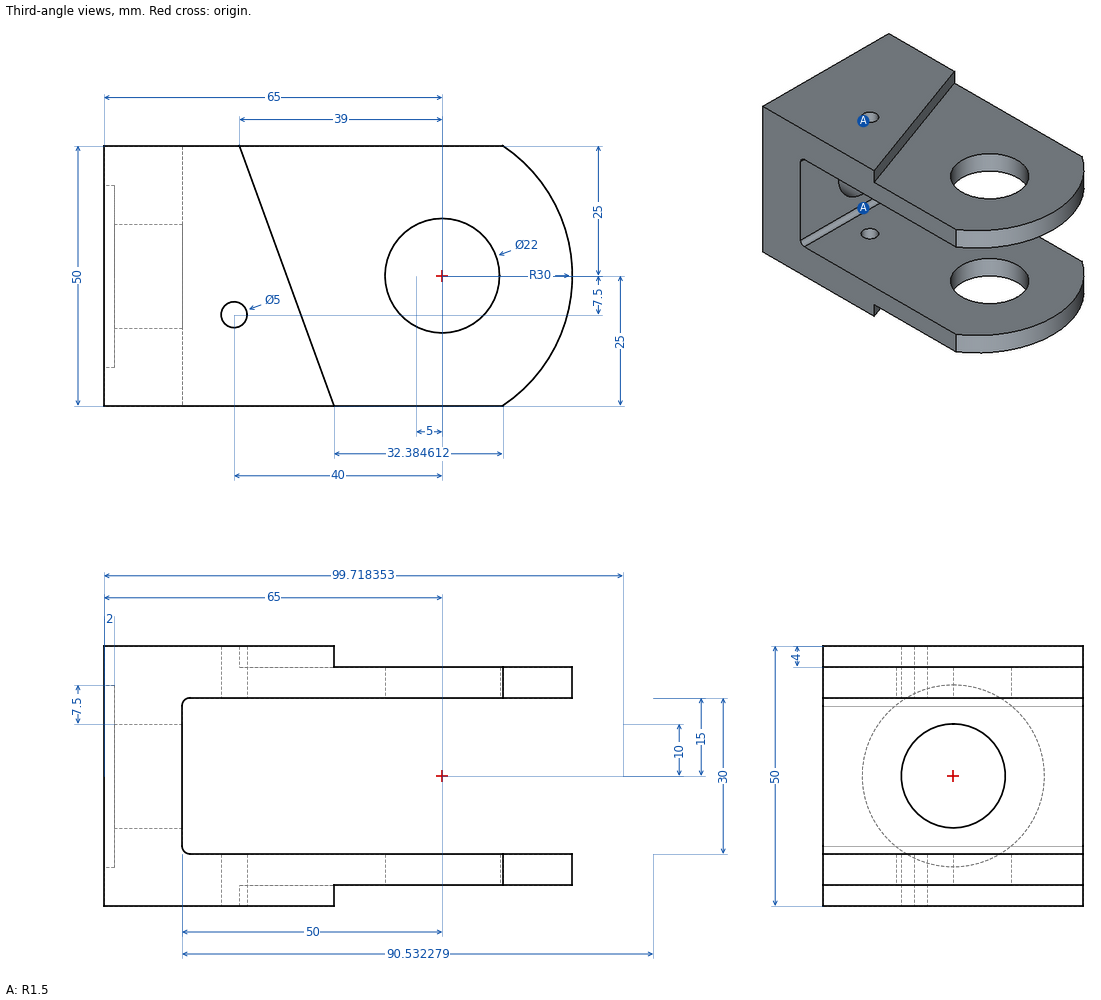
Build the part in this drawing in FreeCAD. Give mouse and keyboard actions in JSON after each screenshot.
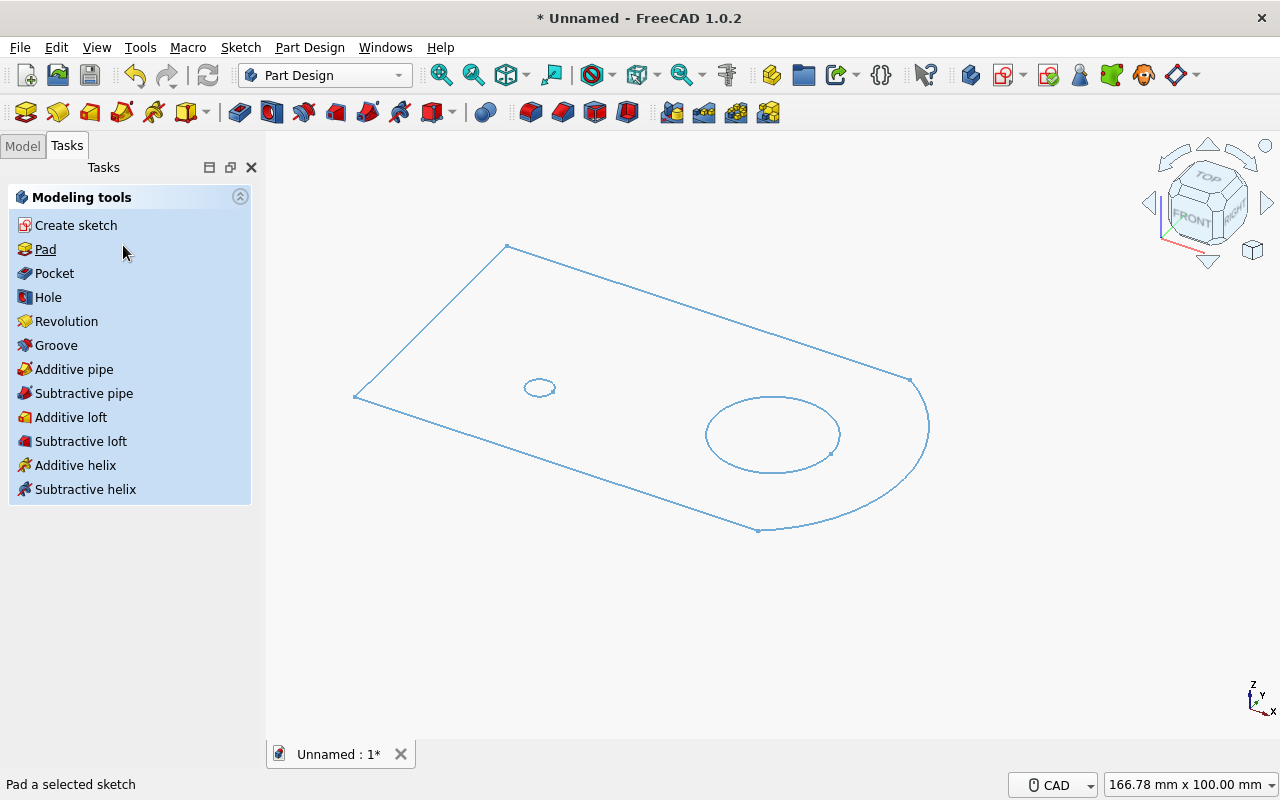
{"action": "left_click", "coordinate": [26, 112]}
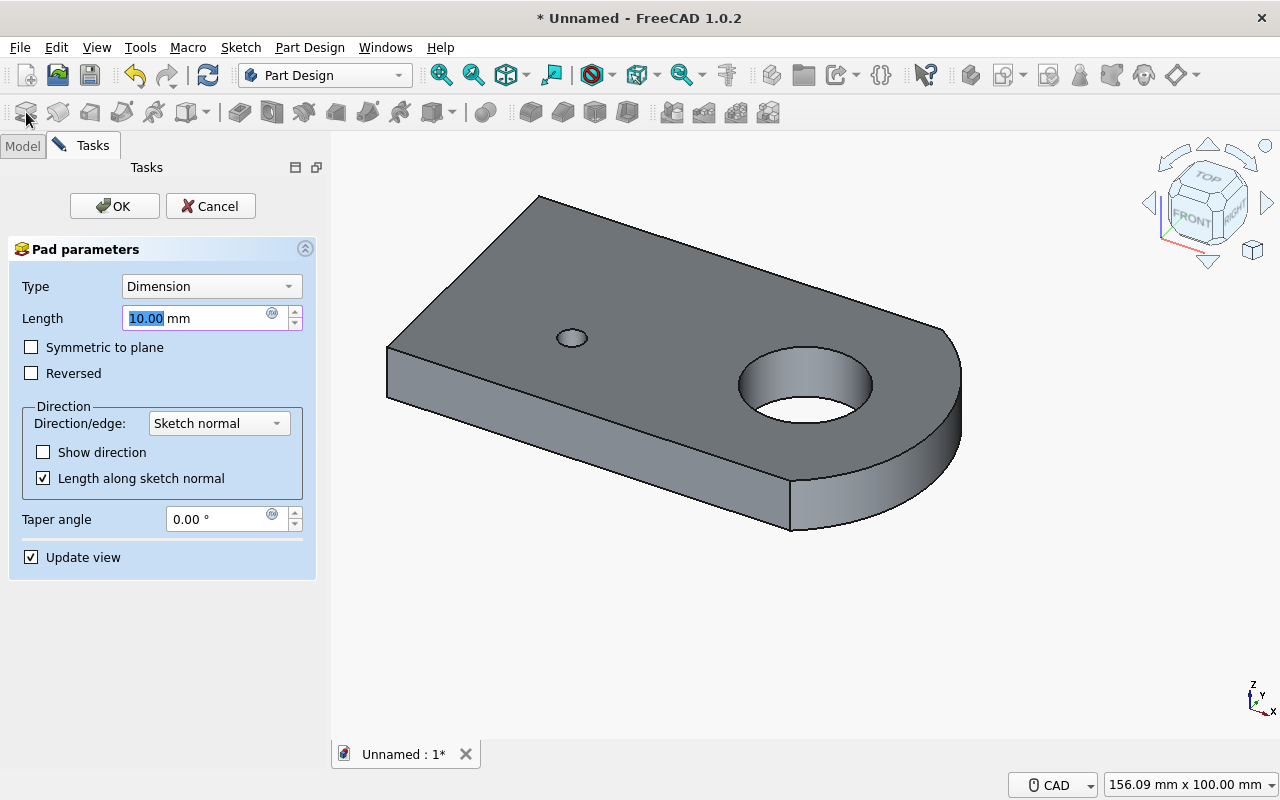
{"action": "type", "text": "50"}
{"action": "key", "text": "Tab"}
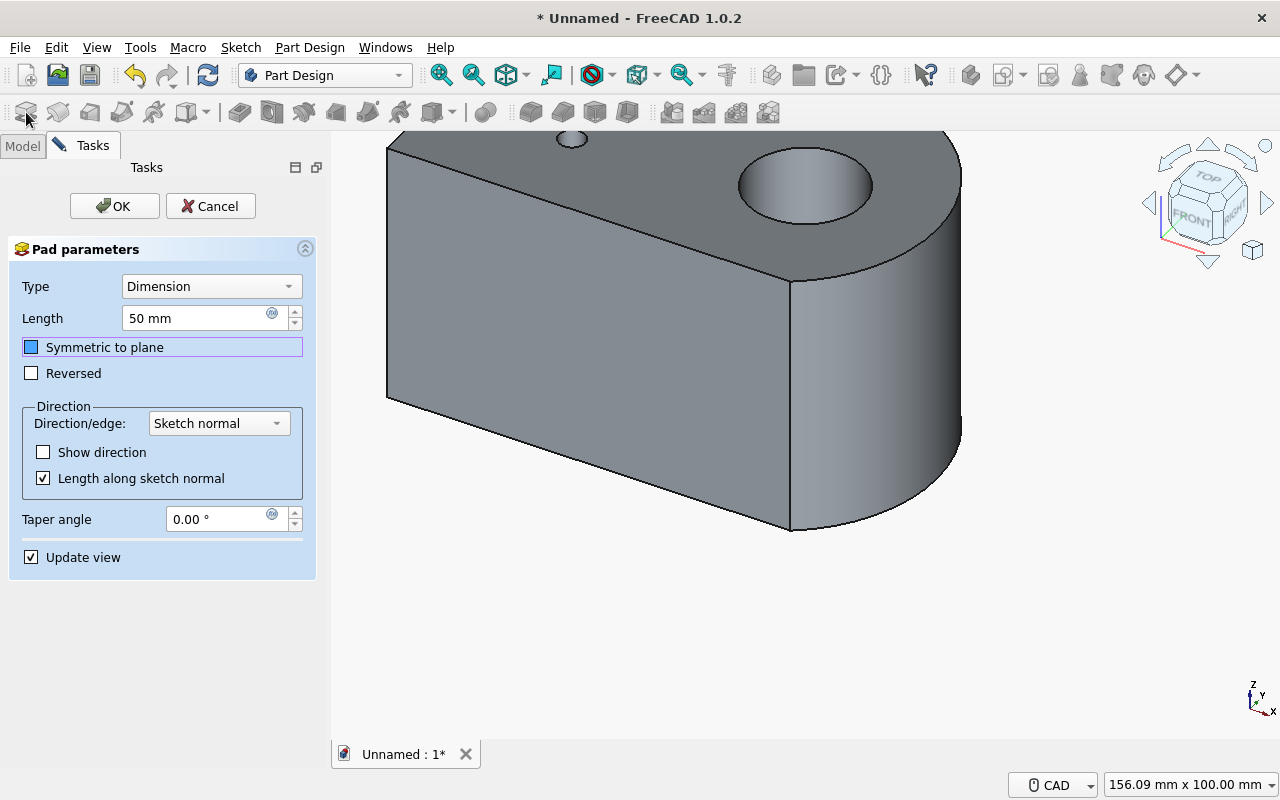
{"action": "left_click", "coordinate": [30, 347]}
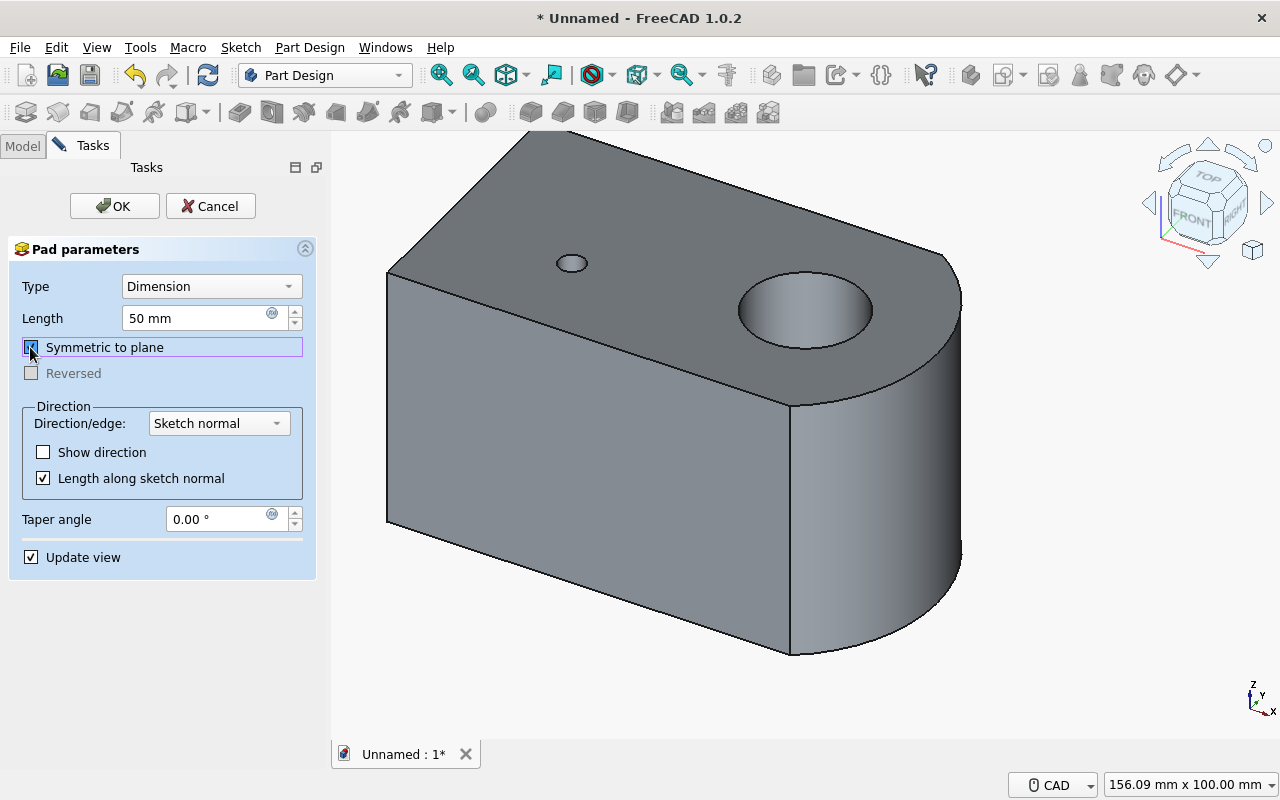
{"action": "left_click", "coordinate": [115, 206]}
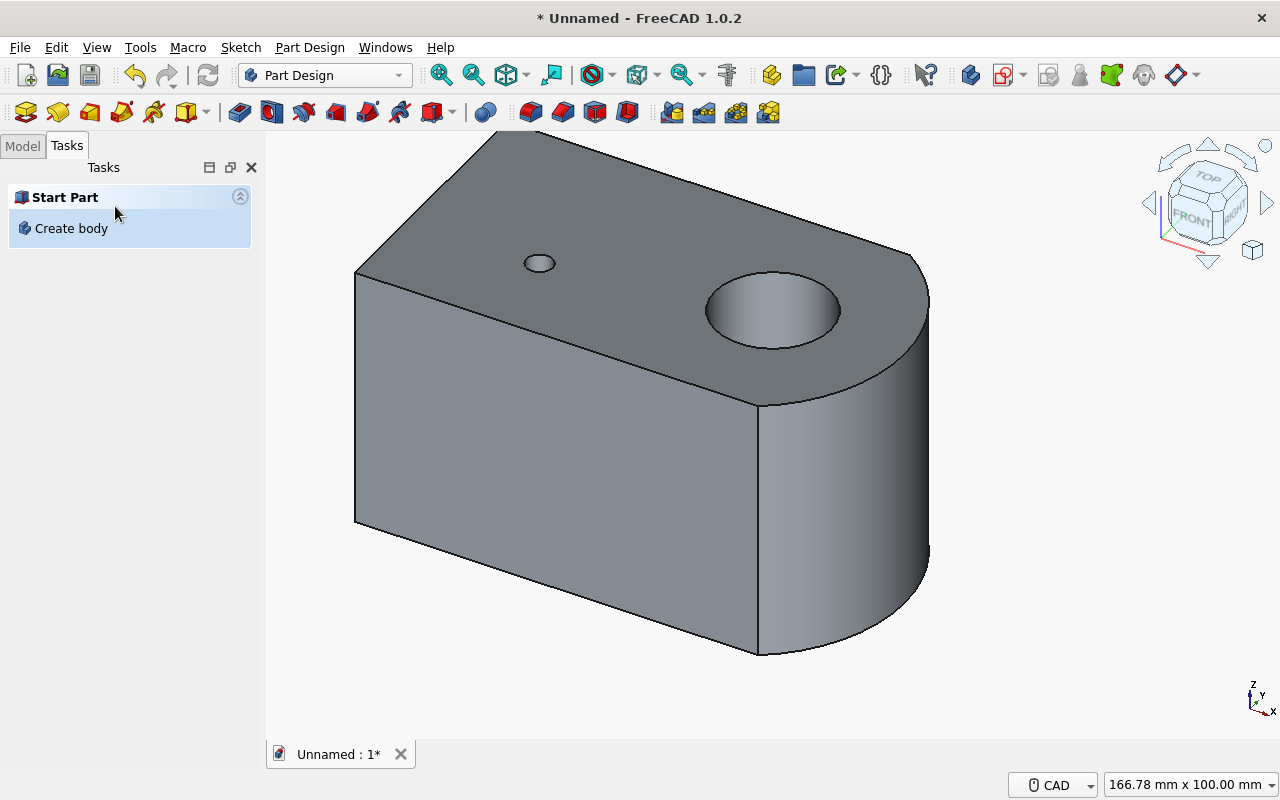
{"action": "left_click", "coordinate": [442, 76]}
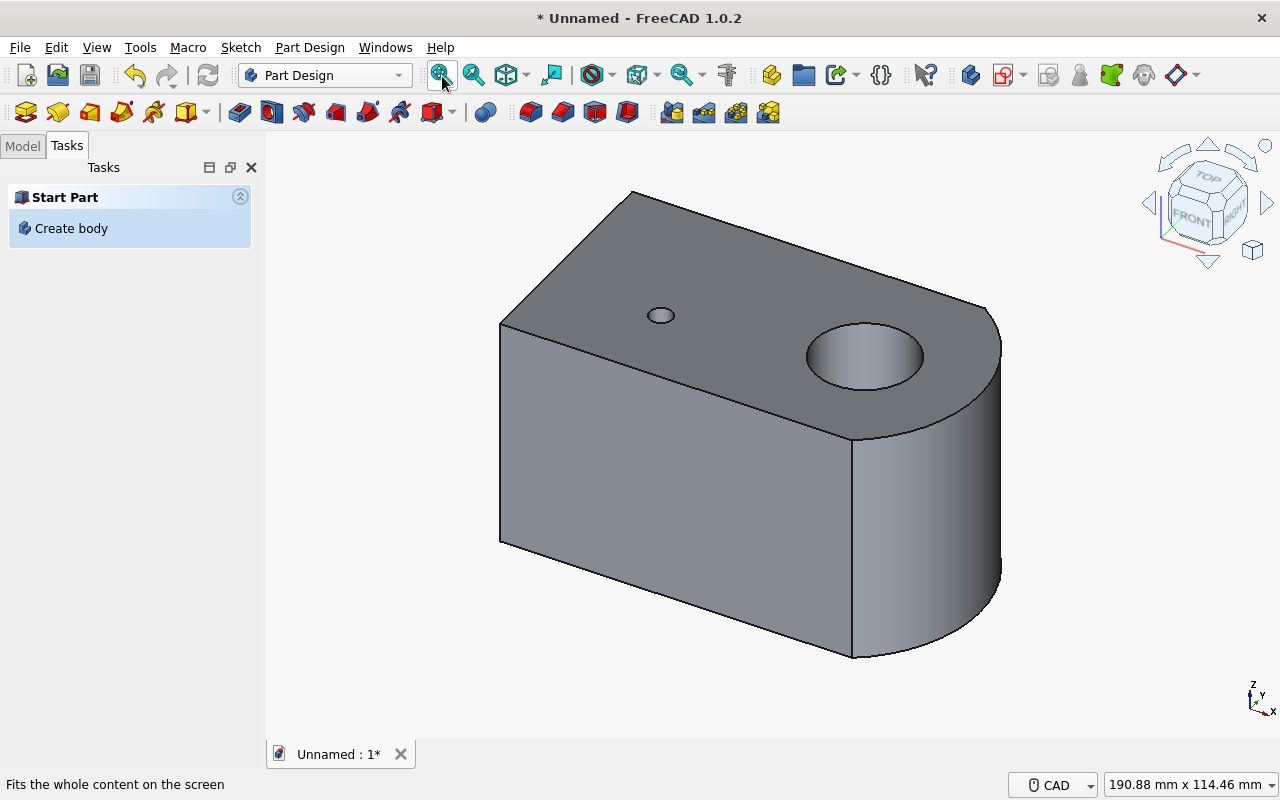
{"action": "key", "text": "4"}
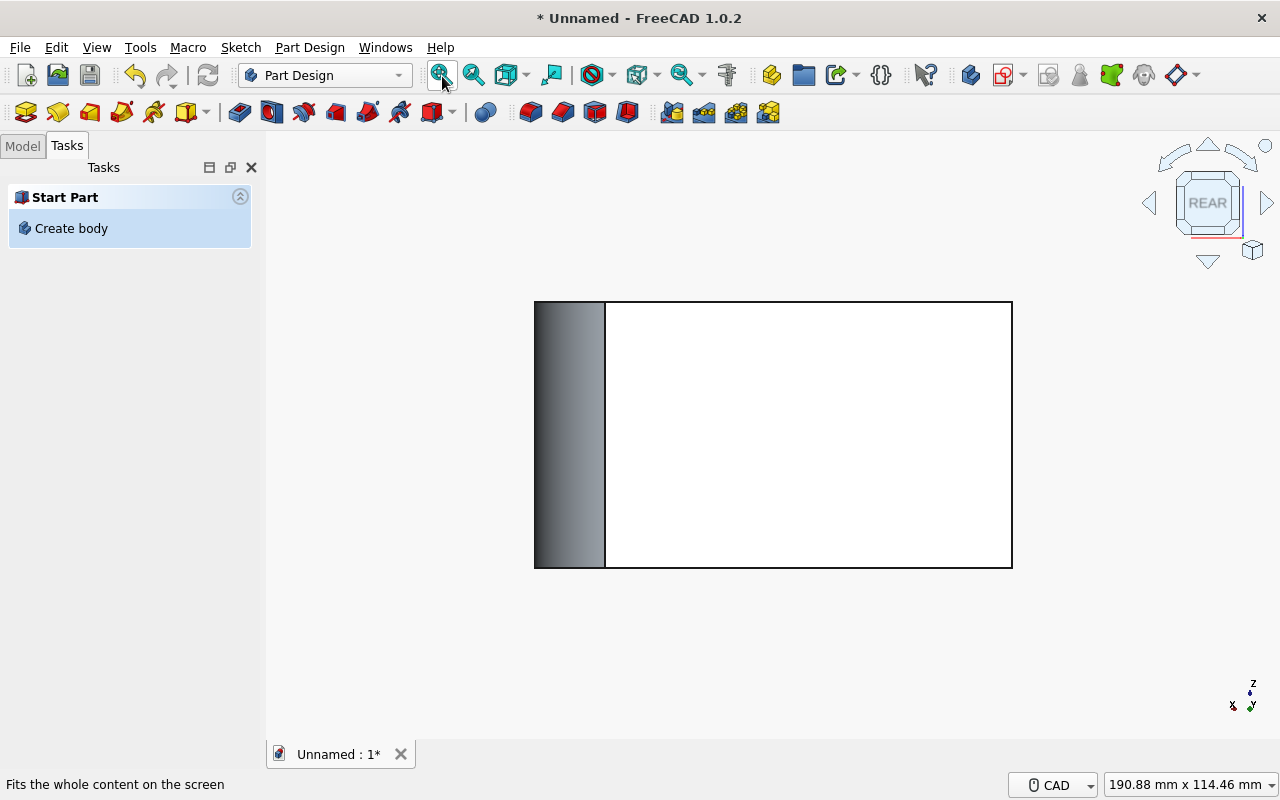
{"action": "left_click", "coordinate": [751, 434]}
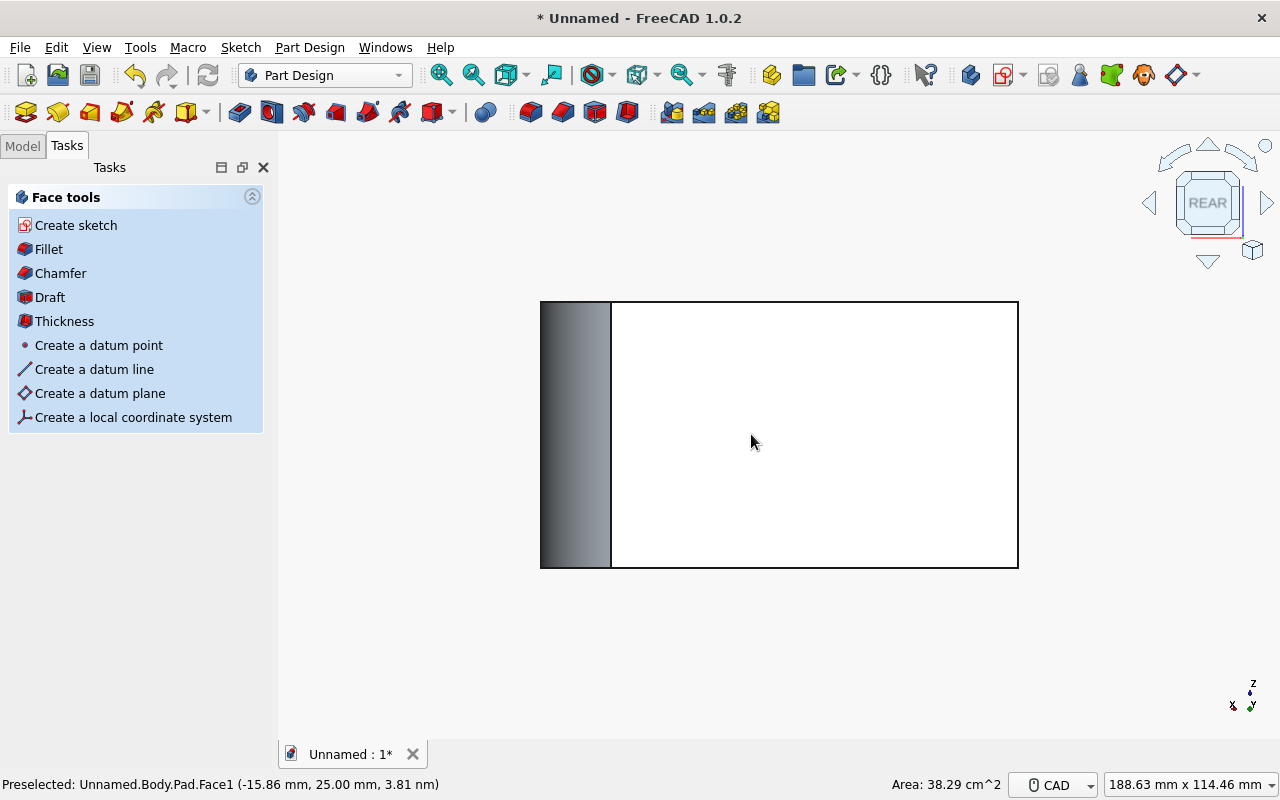
{"action": "left_click", "coordinate": [1004, 76]}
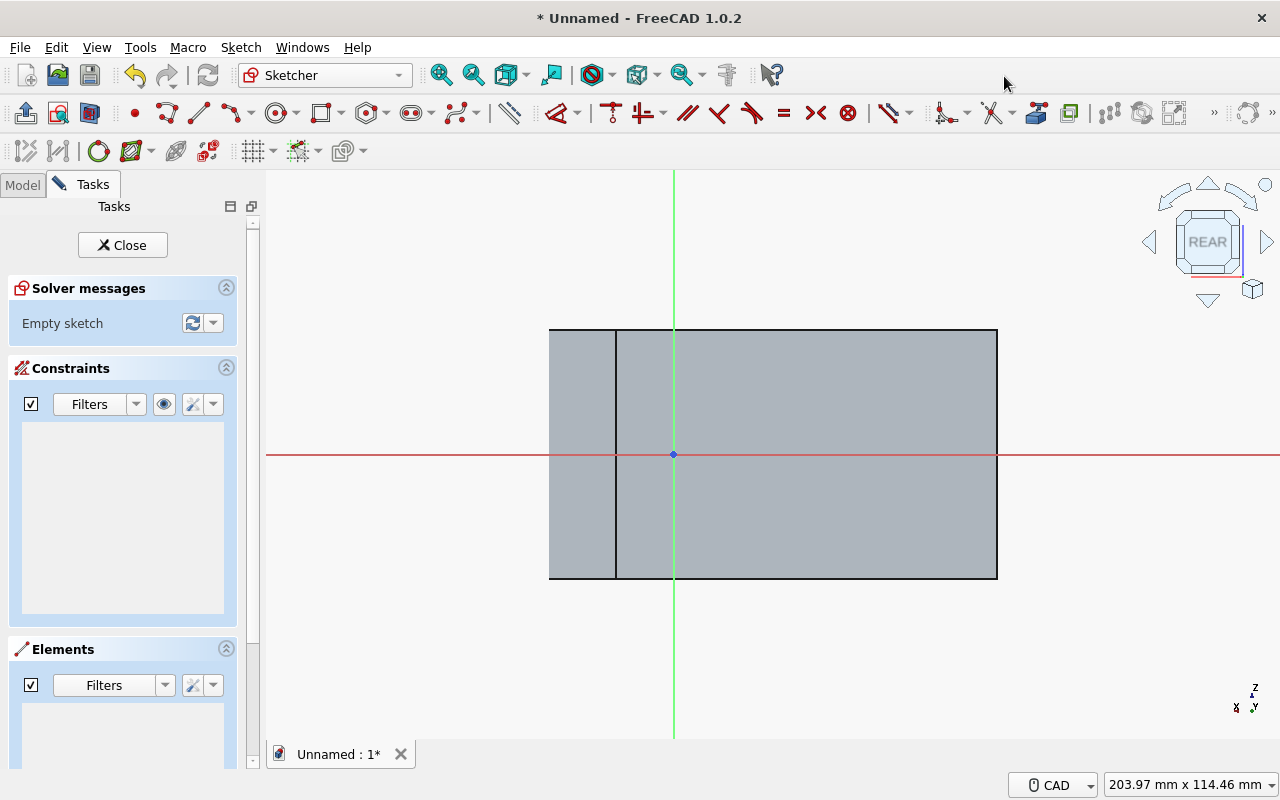
{"action": "left_click", "coordinate": [322, 114]}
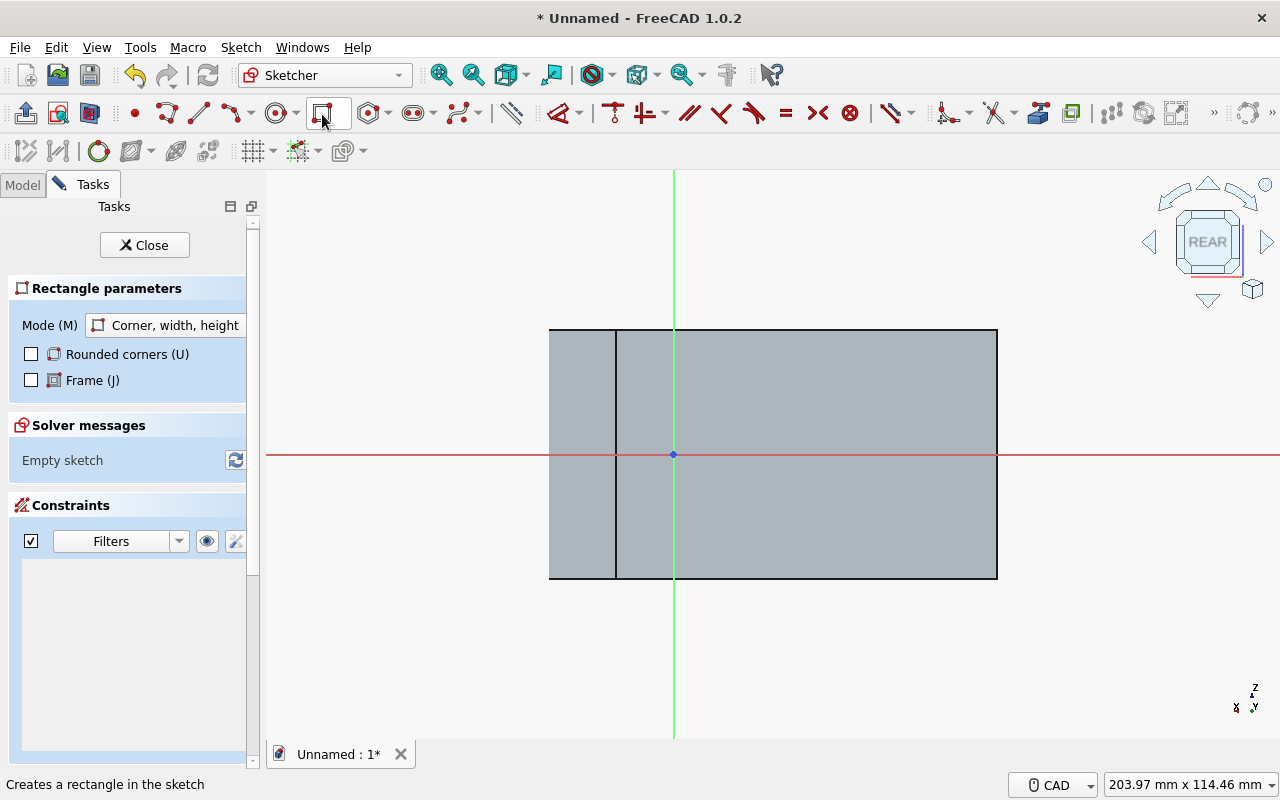
{"action": "left_click", "coordinate": [472, 380]}
{"action": "left_click", "coordinate": [922, 529]}
{"action": "key", "text": "Escape"}